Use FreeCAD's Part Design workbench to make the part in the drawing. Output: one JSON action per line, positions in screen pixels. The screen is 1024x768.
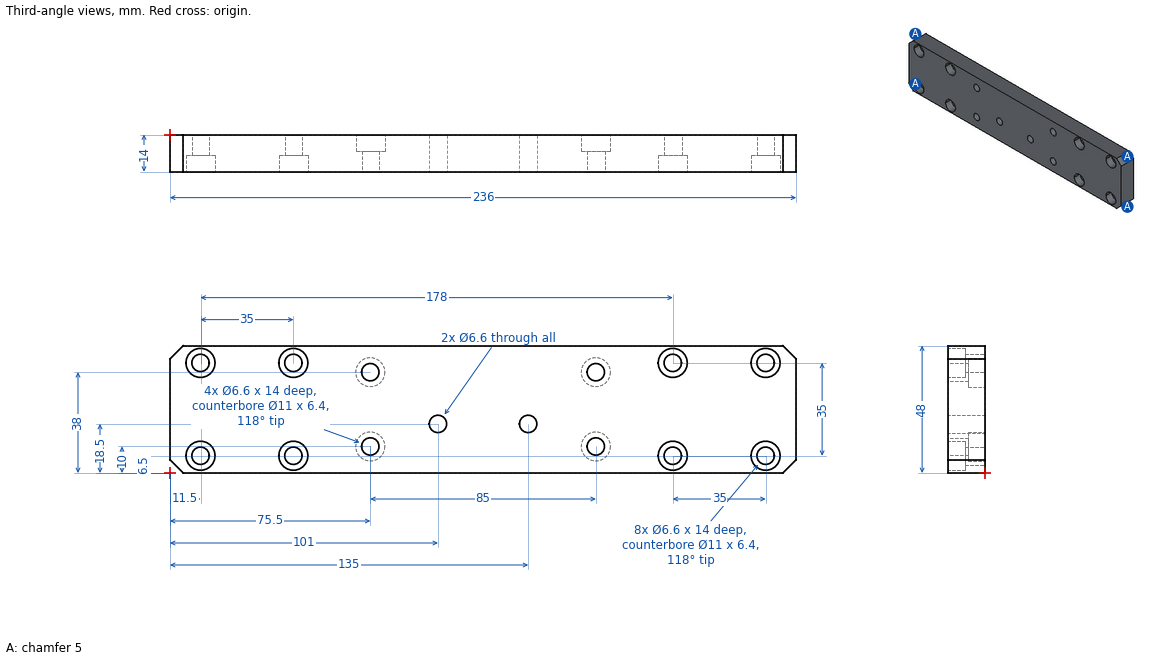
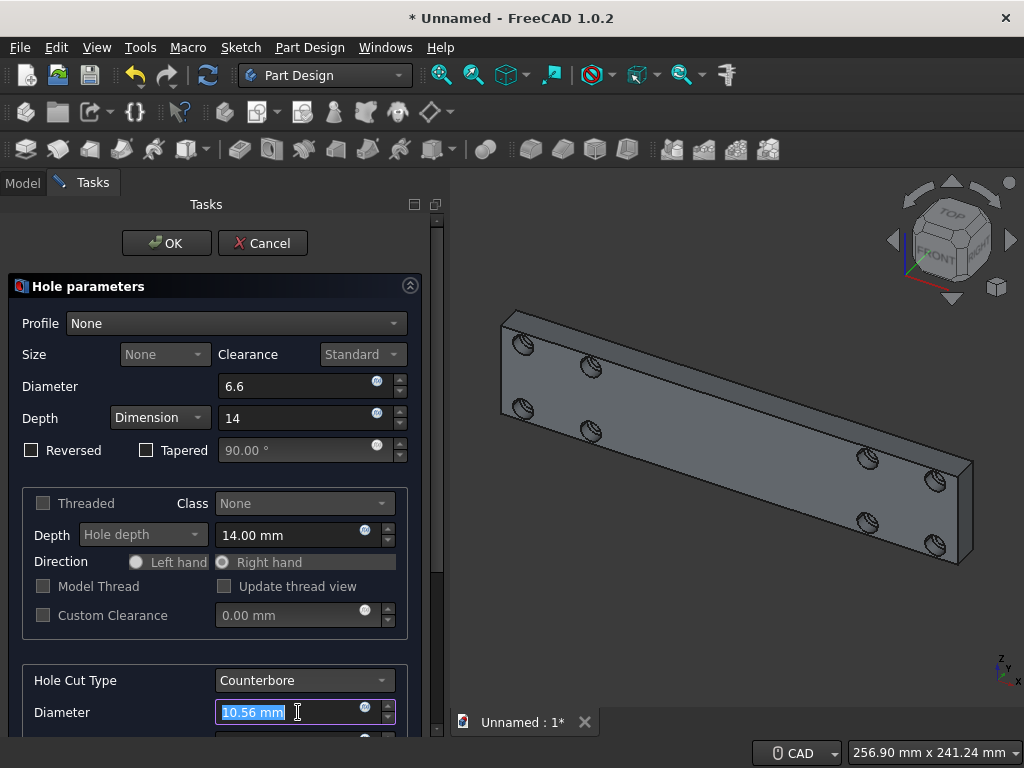
{"action": "type", "text": "11"}
{"action": "key", "text": "Tab"}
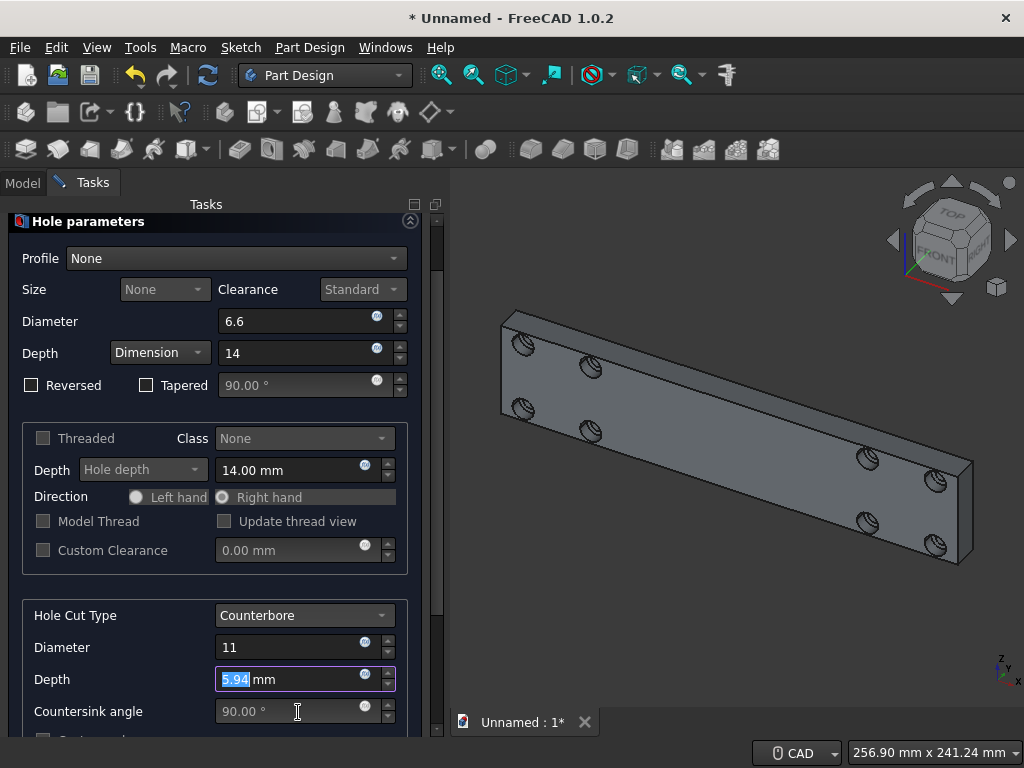
{"action": "type", "text": "6.4"}
{"action": "key", "text": "Tab"}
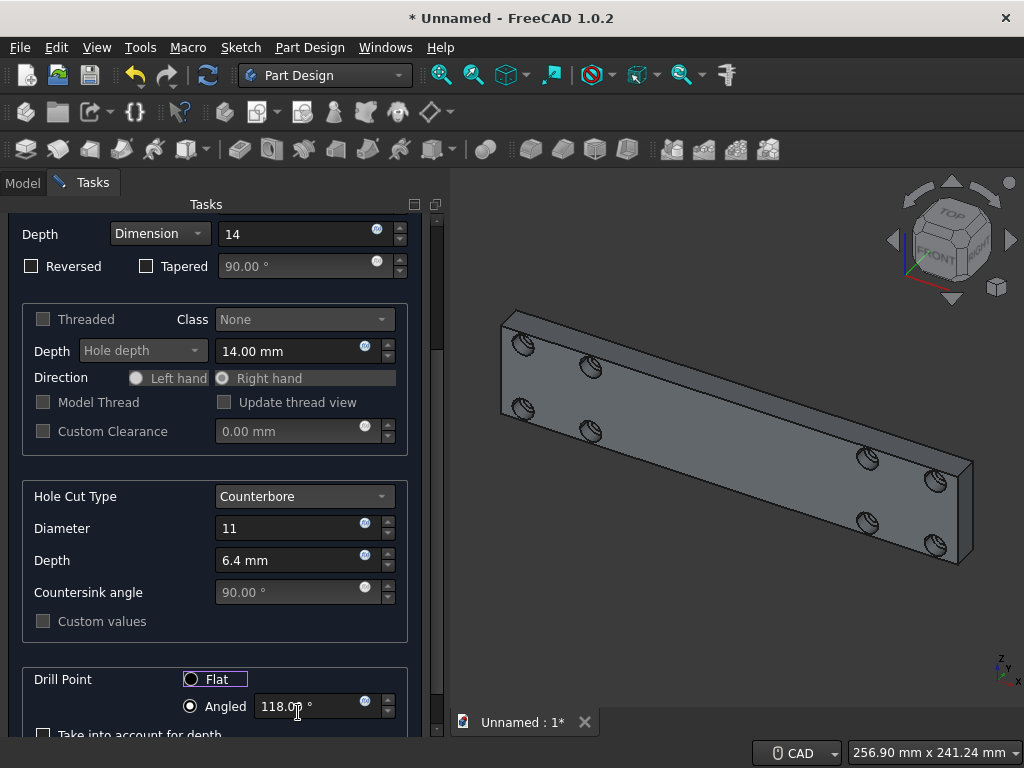
{"action": "scroll", "coordinate": [437, 475], "scroll_direction": "up", "scroll_amount": 4}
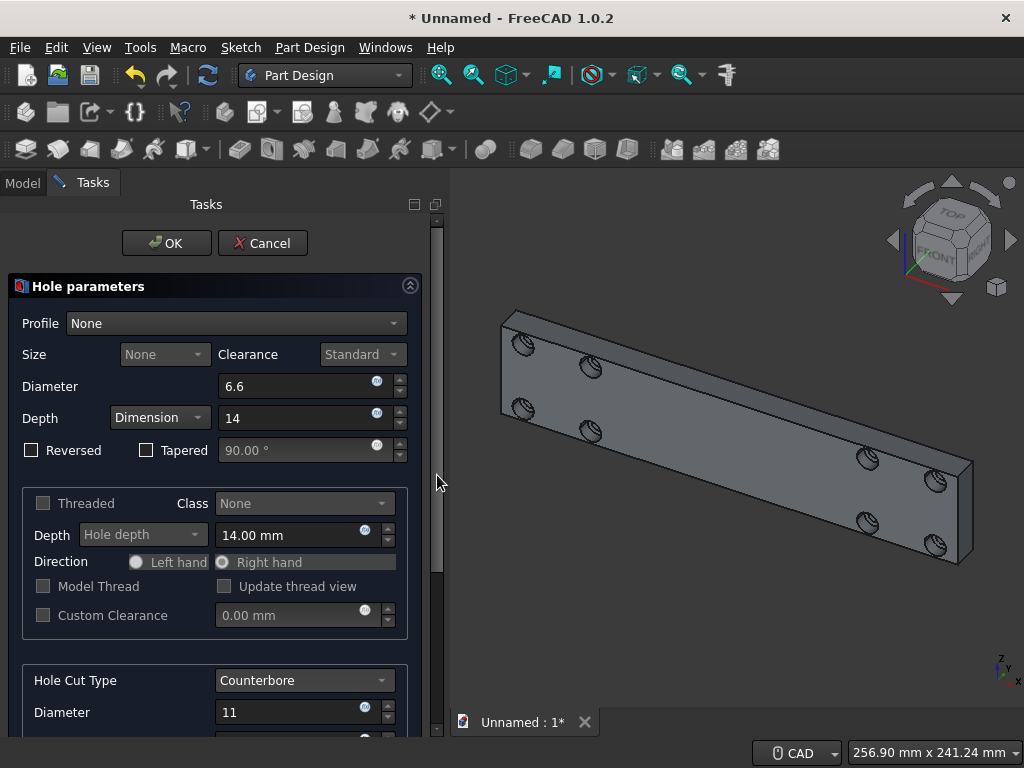
{"action": "left_click", "coordinate": [167, 243]}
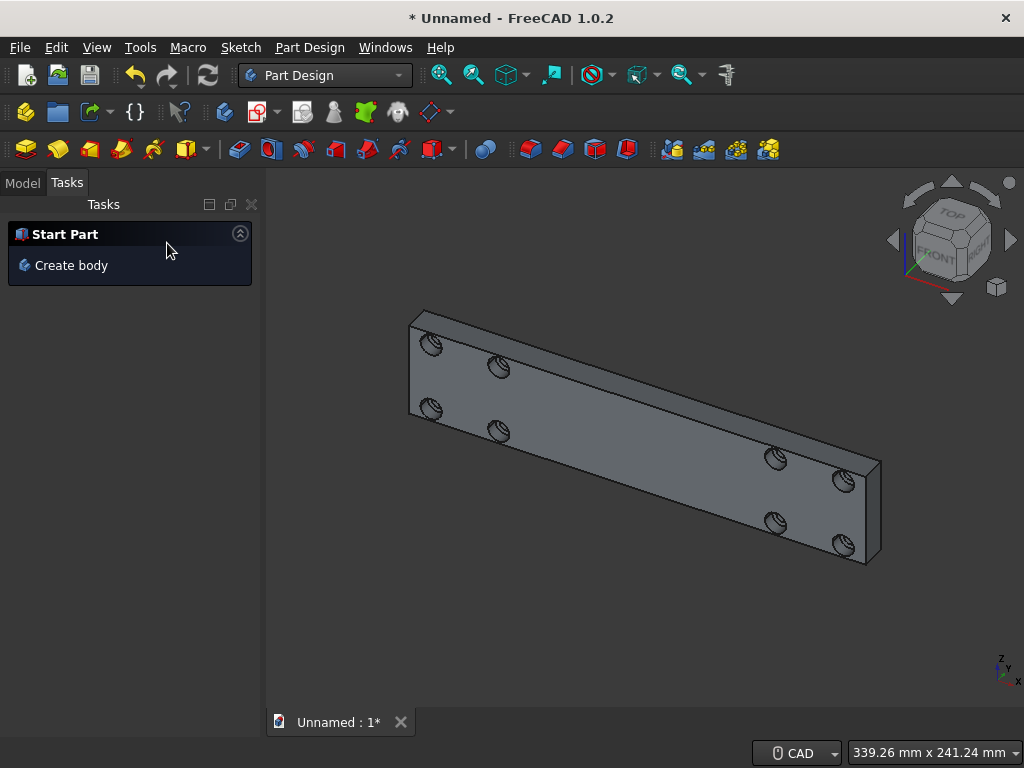
{"action": "left_click", "coordinate": [873, 468]}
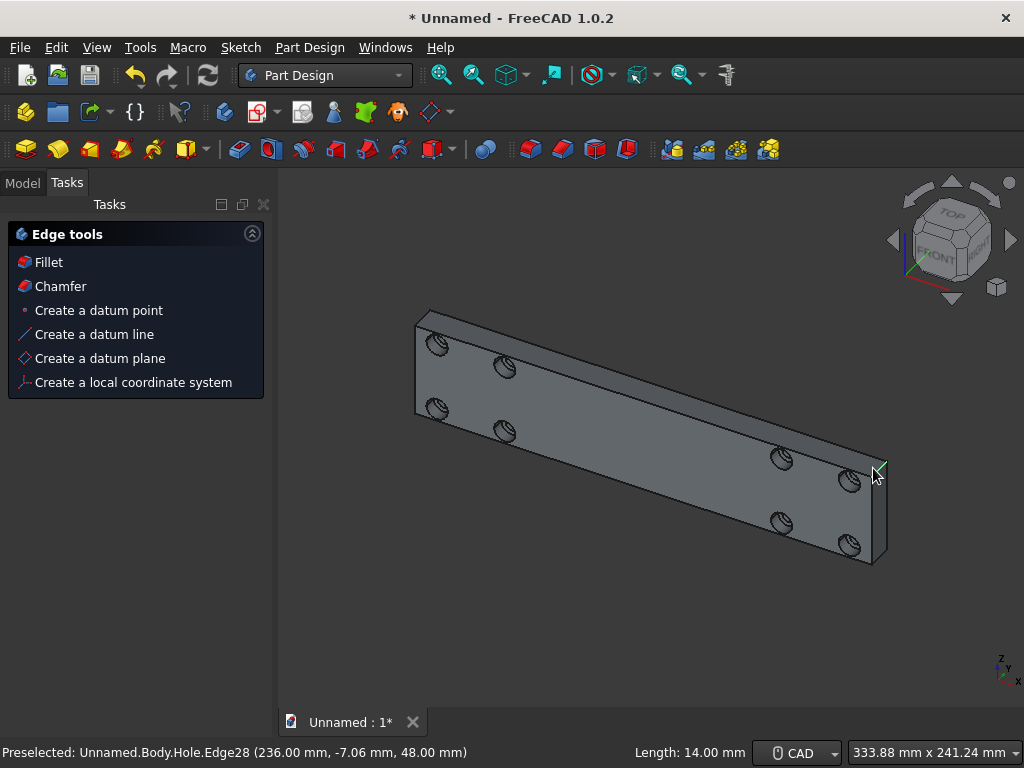
{"action": "key", "text": "0"}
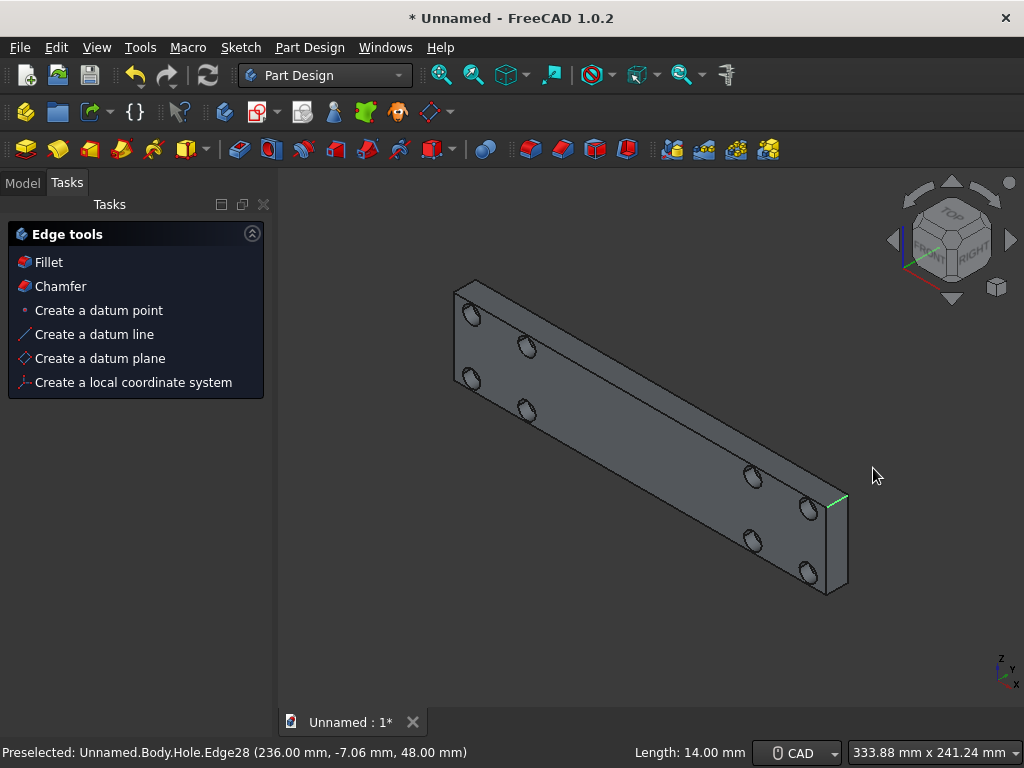
{"action": "key", "text": "2"}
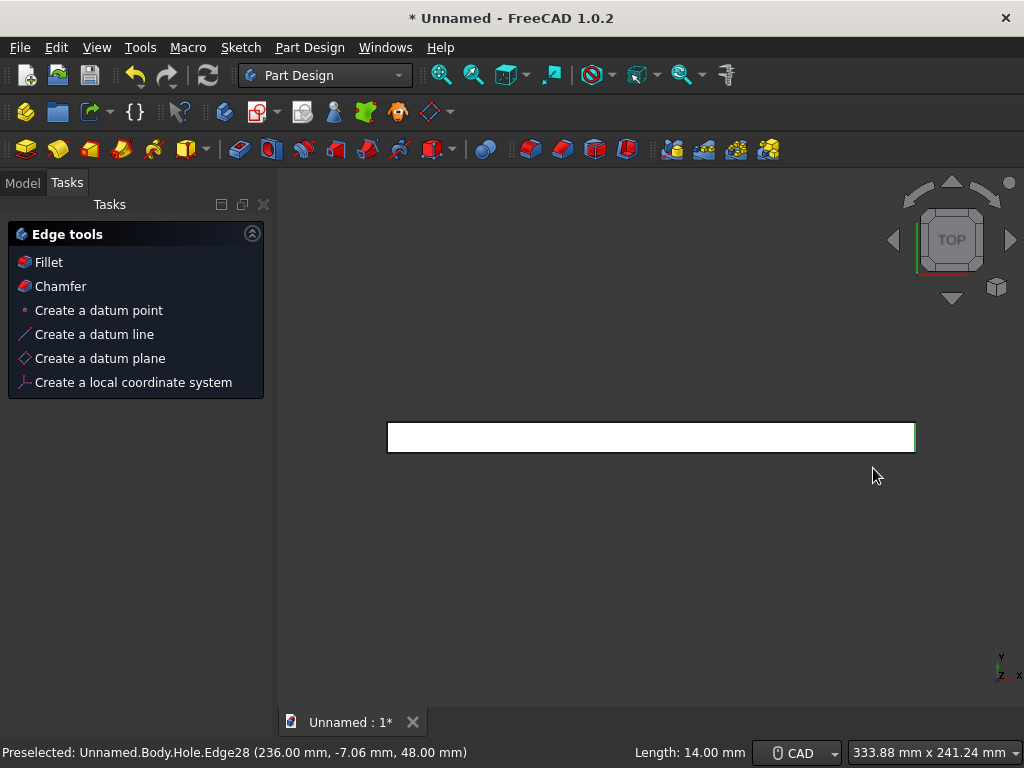
{"action": "left_click", "coordinate": [387, 437], "text": "ctrl"}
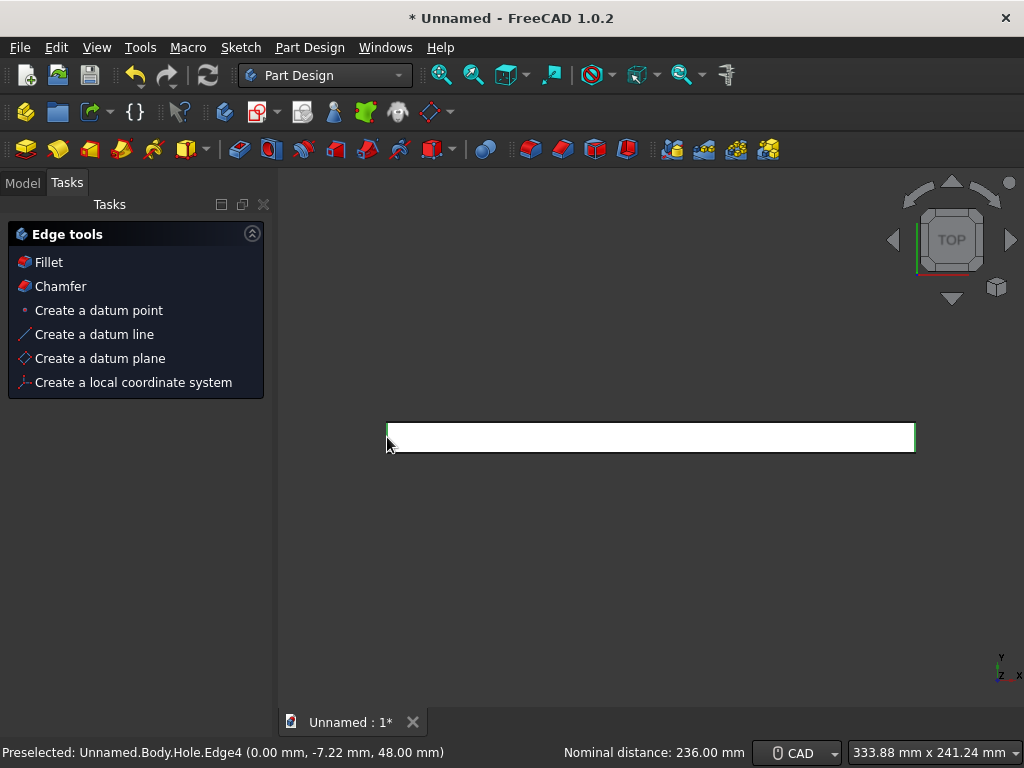
{"action": "key", "text": "1"}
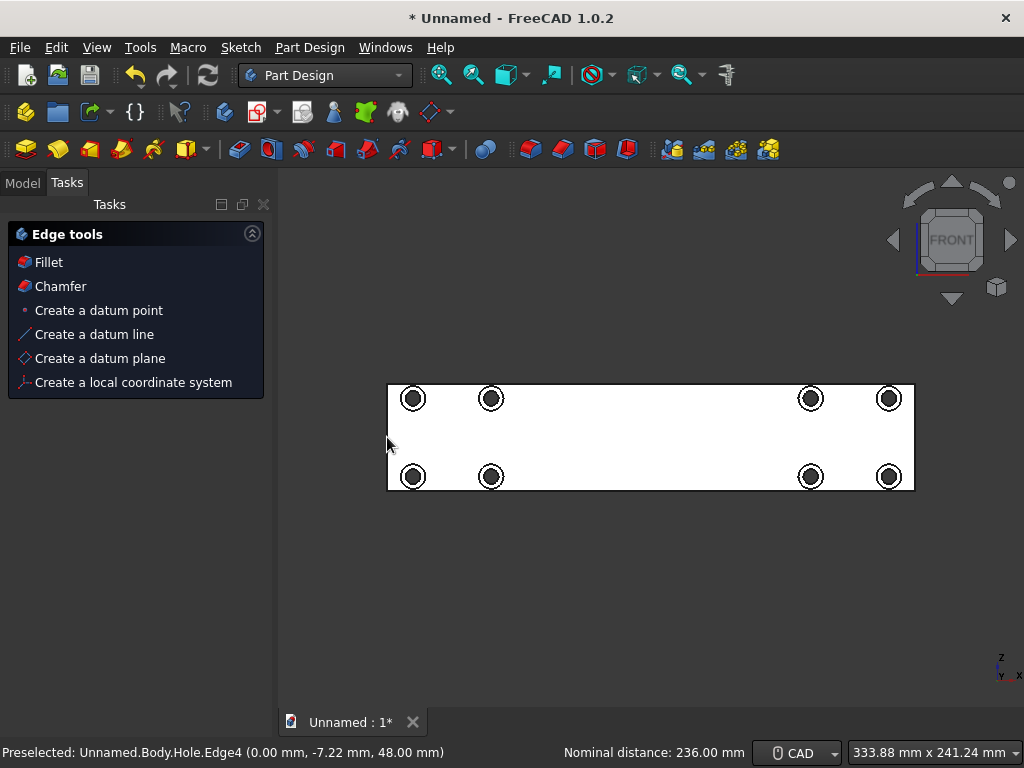
{"action": "key", "text": "3"}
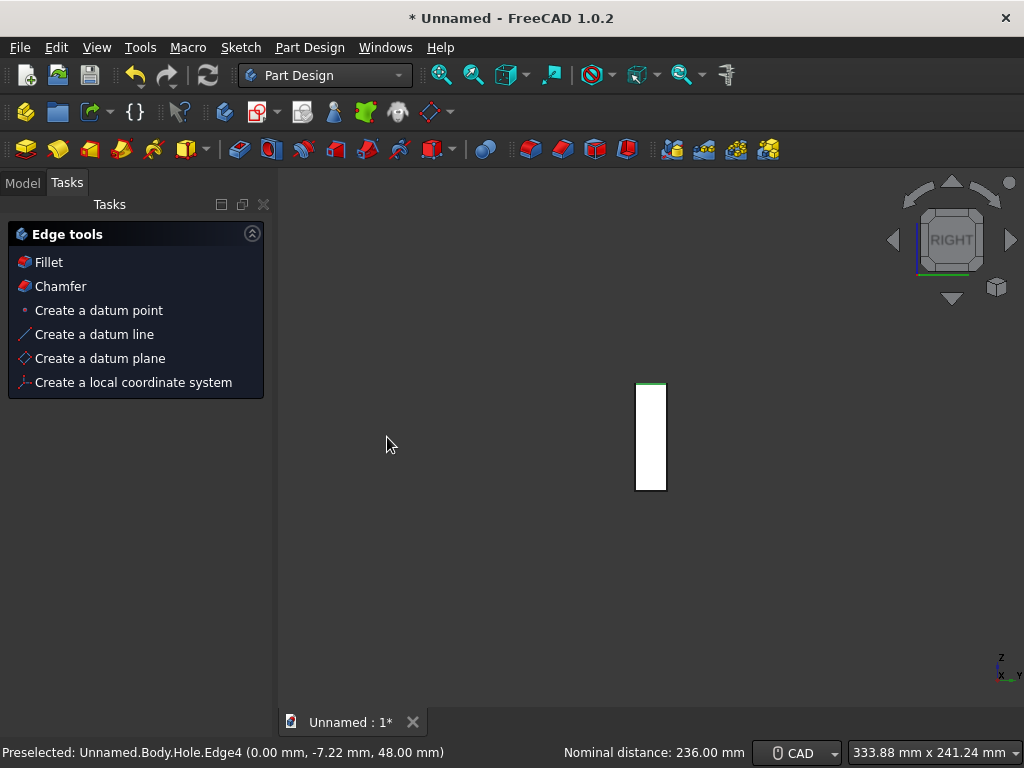
{"action": "left_click", "coordinate": [442, 76]}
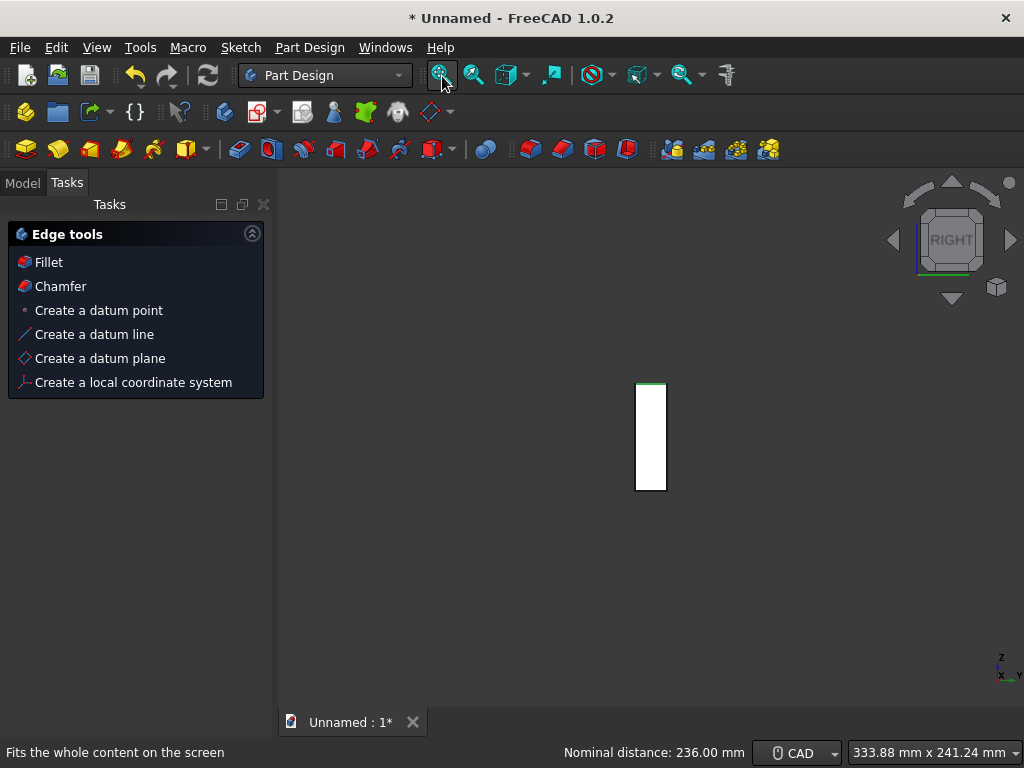
{"action": "left_click", "coordinate": [651, 490], "text": "ctrl"}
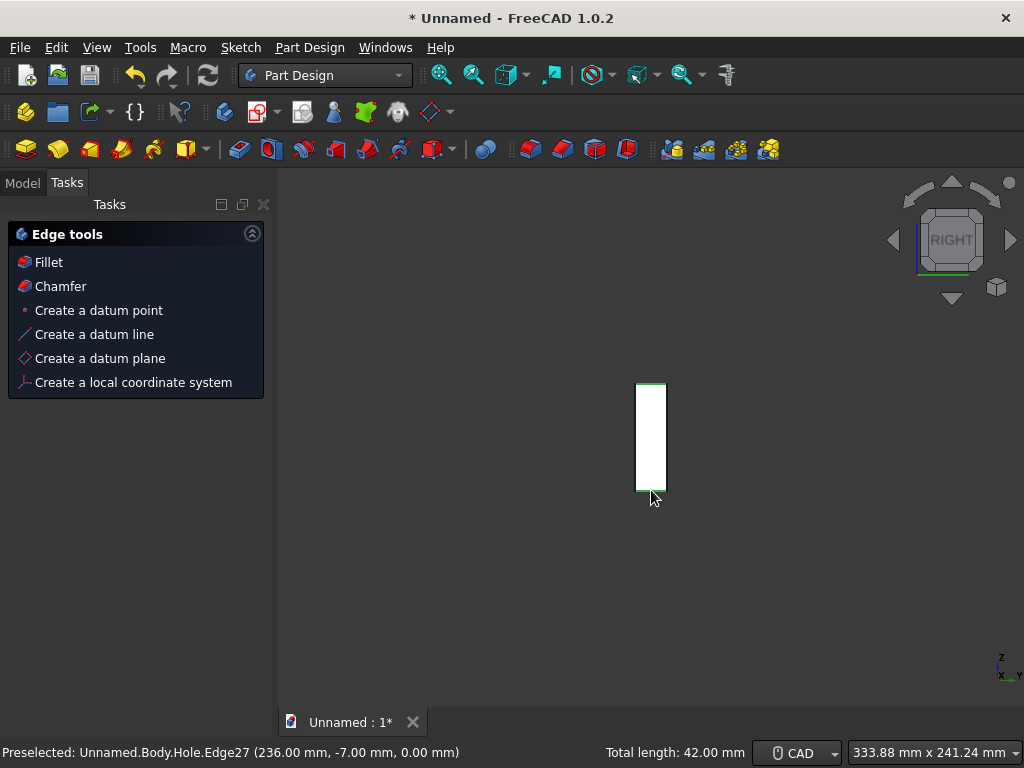
{"action": "key", "text": "5"}